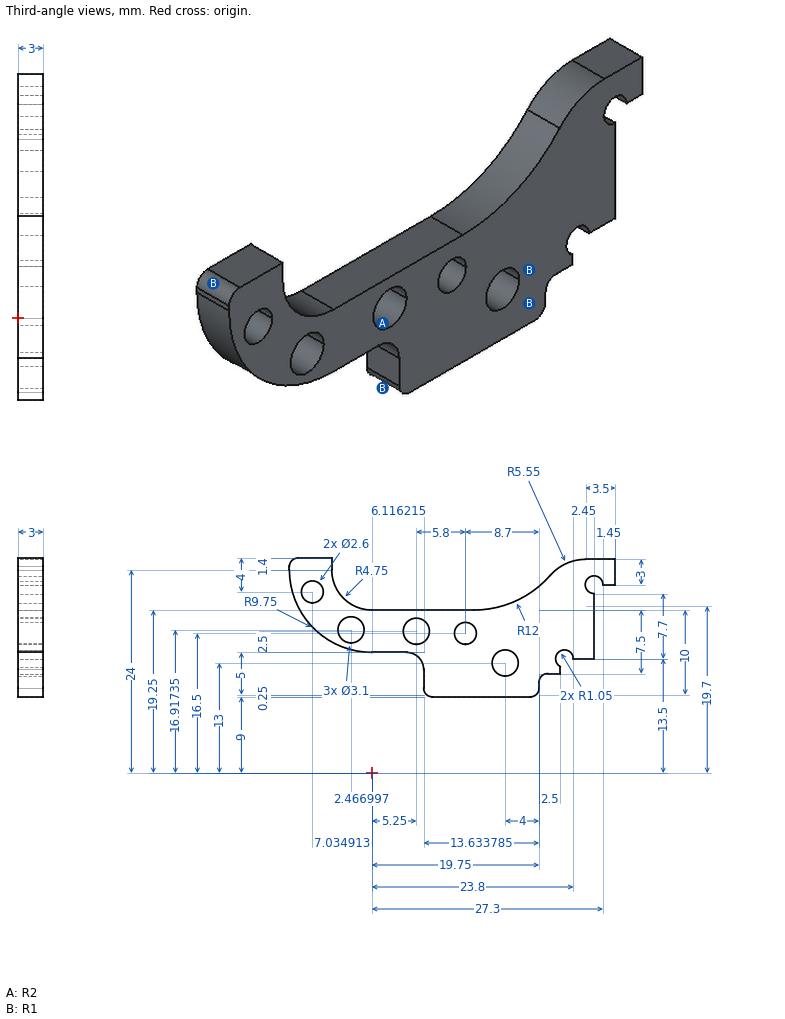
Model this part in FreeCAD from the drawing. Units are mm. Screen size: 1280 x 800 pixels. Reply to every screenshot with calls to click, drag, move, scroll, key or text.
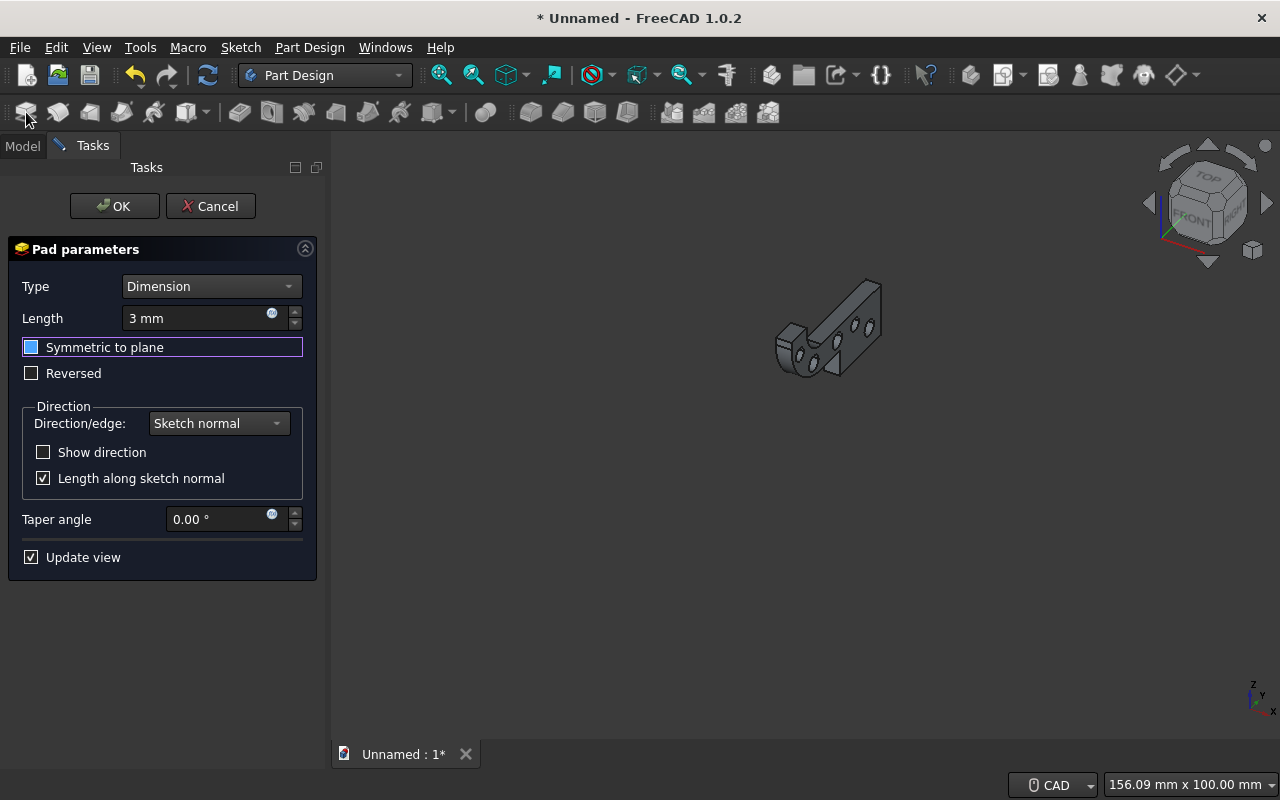
click(115, 206)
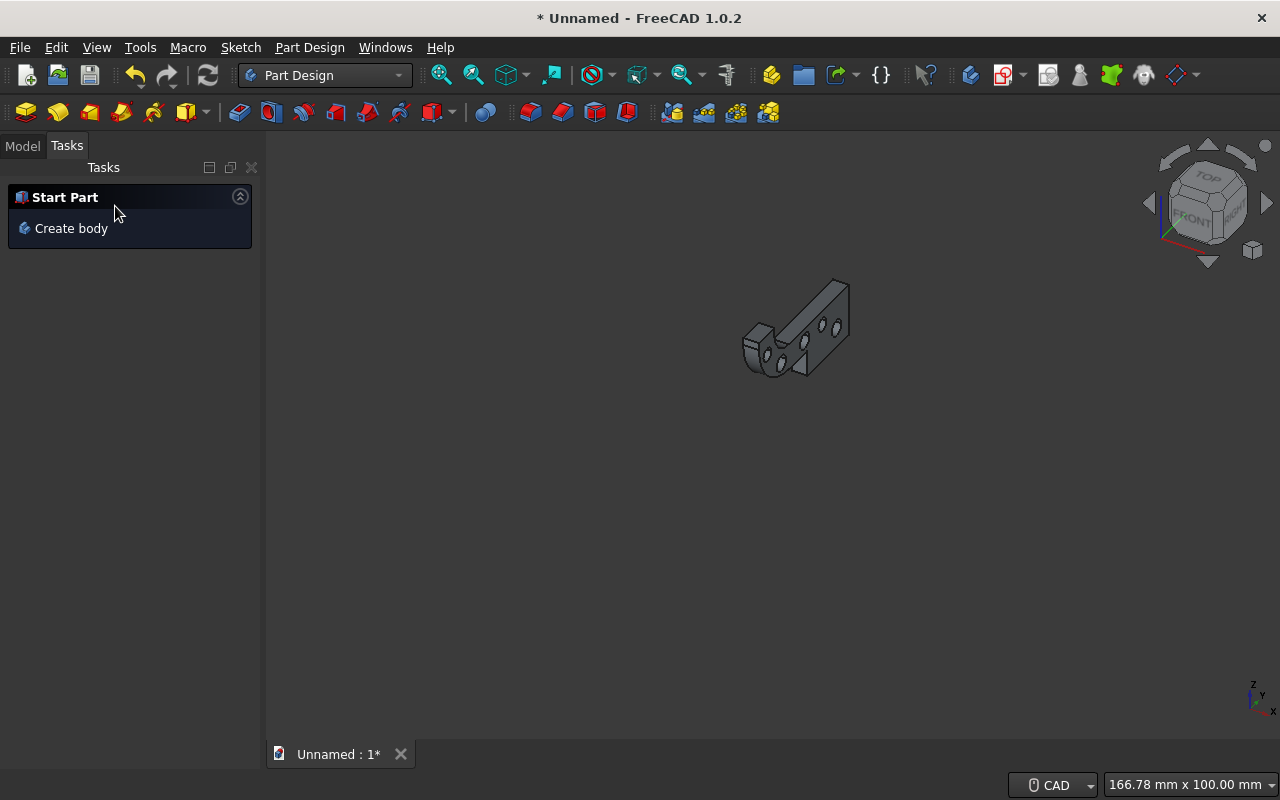
key(v)
key(f)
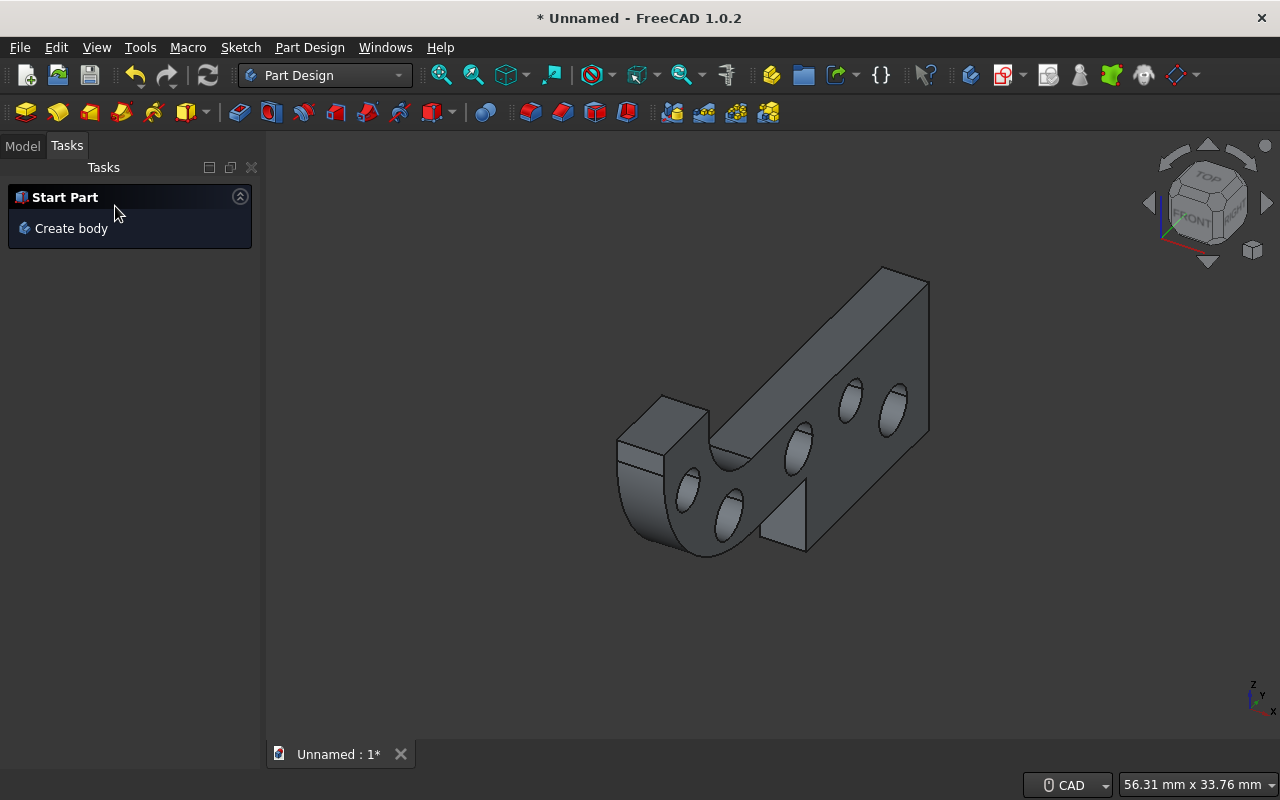
click(834, 472)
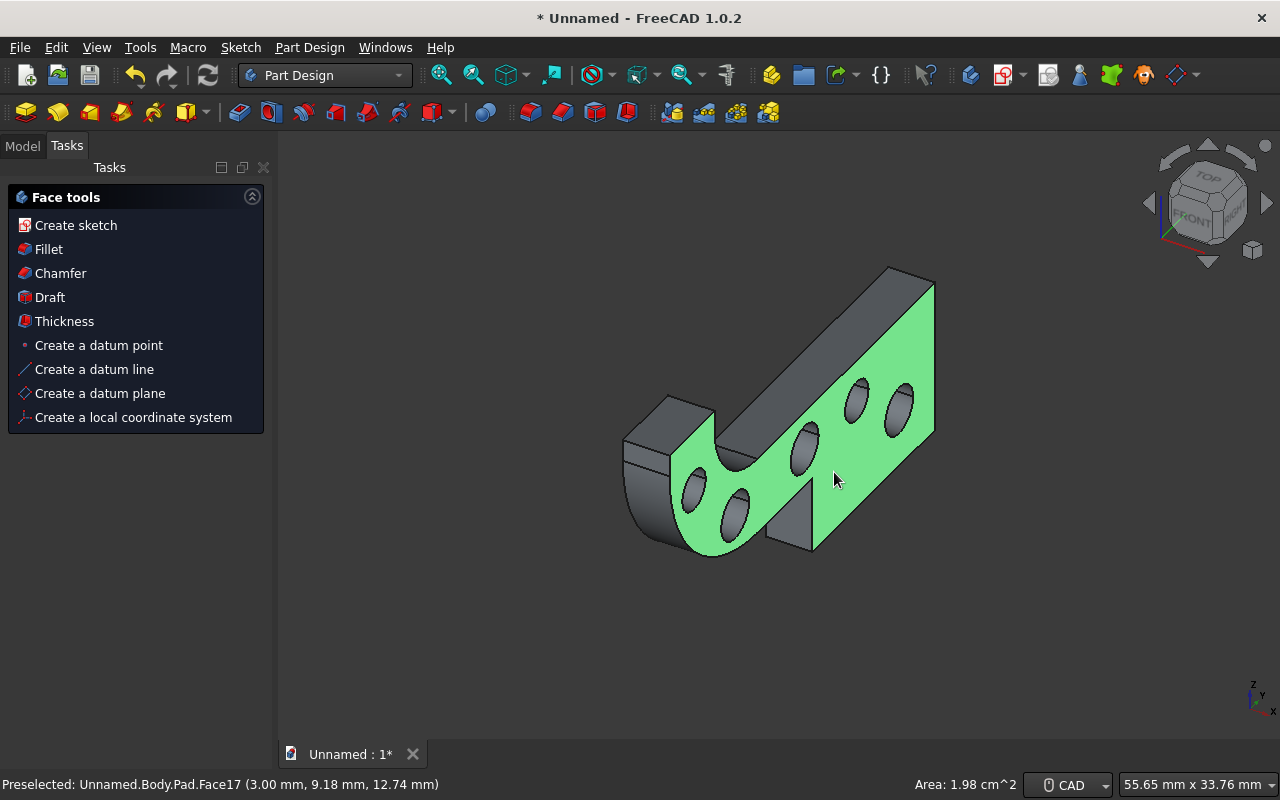
click(1004, 76)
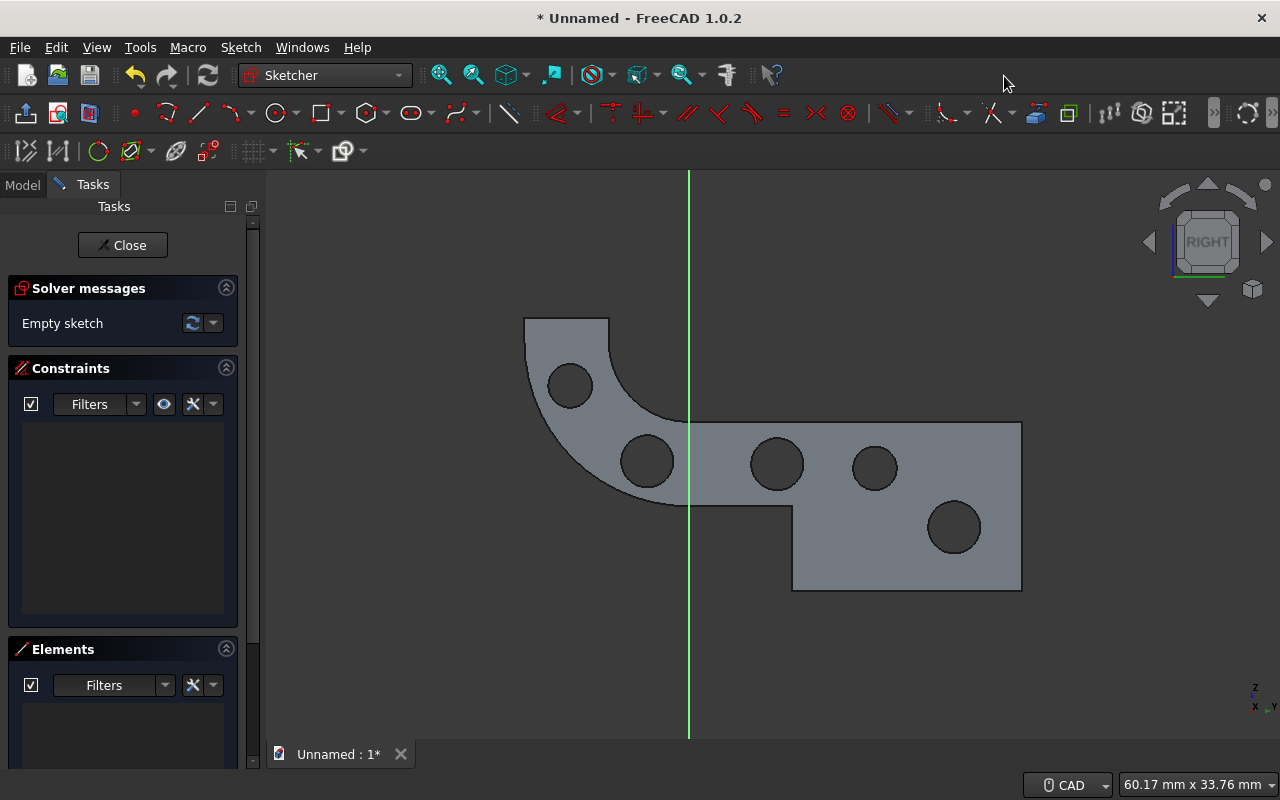
scroll(294, 198, down, 1)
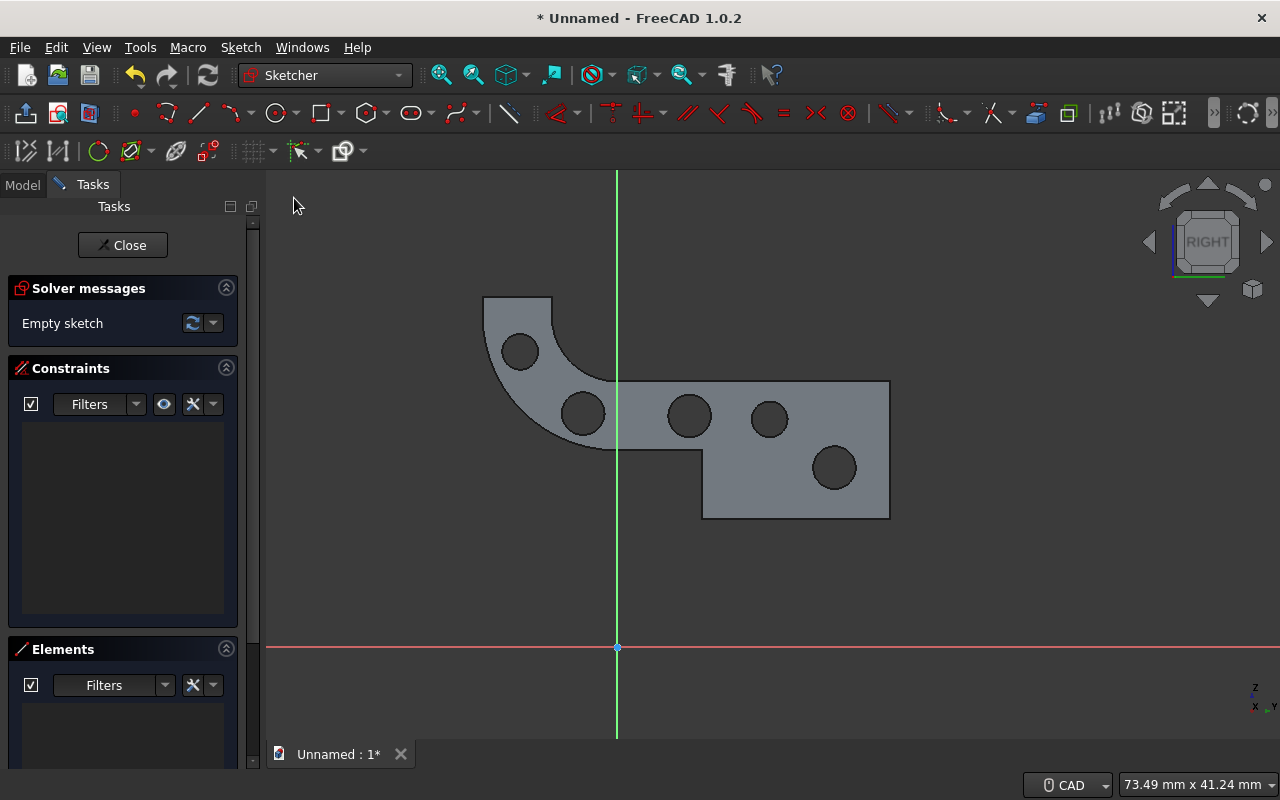
click(168, 114)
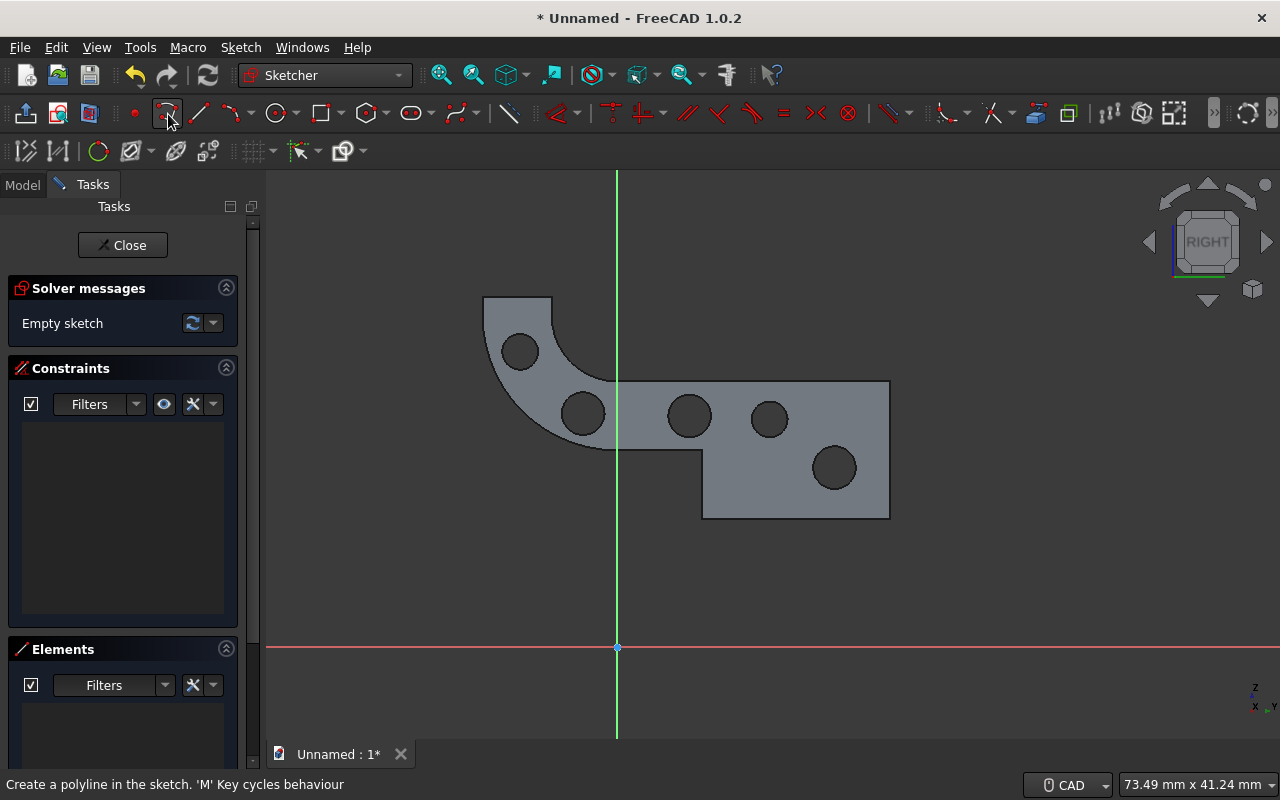
click(946, 461)
click(979, 461)
click(979, 355)
right_click(979, 355)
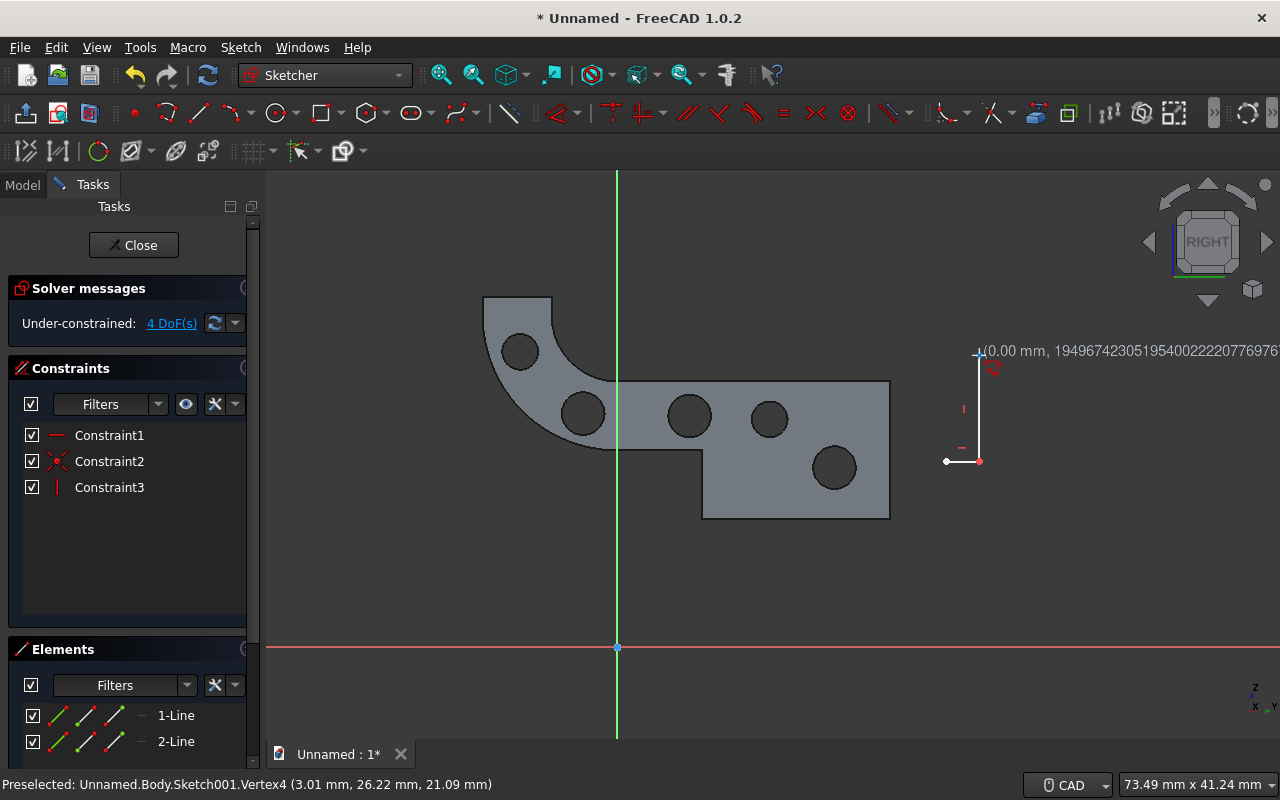
click(994, 340)
click(1014, 340)
click(1014, 299)
click(966, 299)
right_click(966, 299)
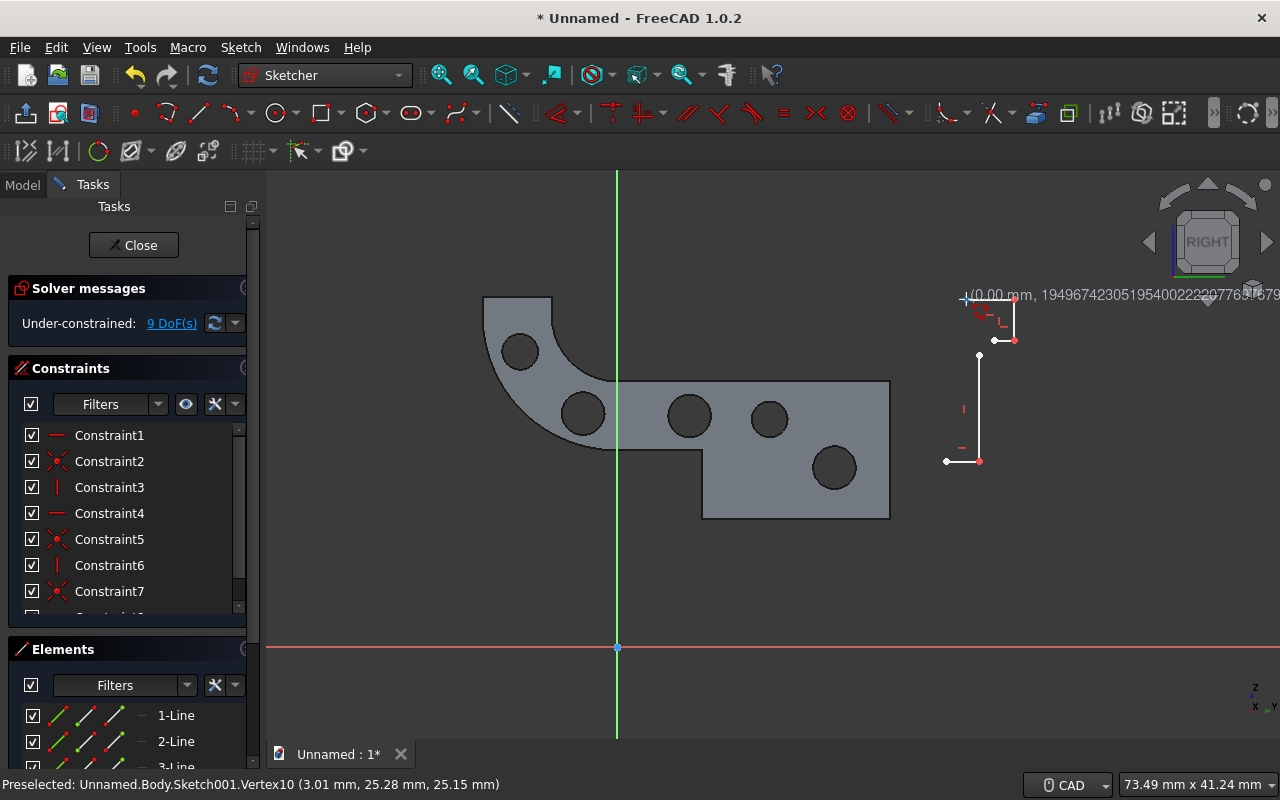
click(783, 381)
click(890, 381)
click(890, 485)
click(924, 485)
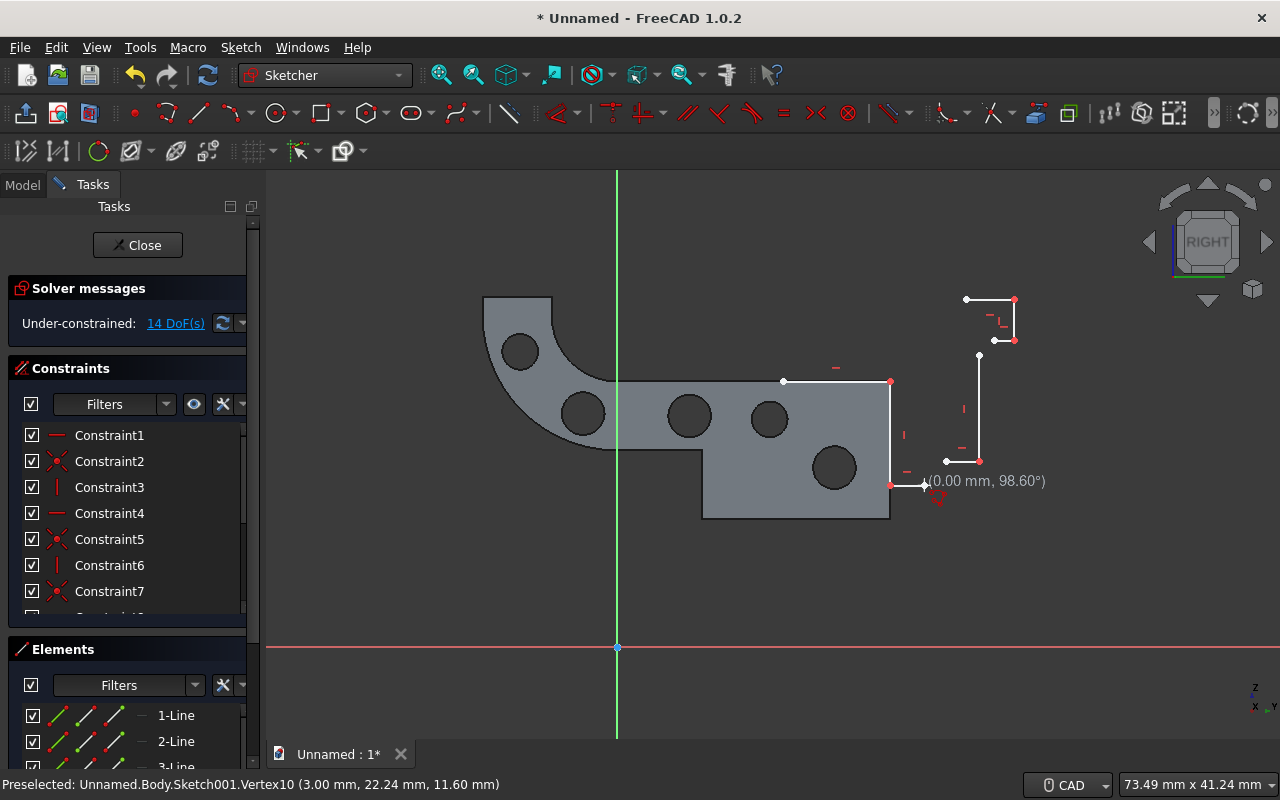
scroll(924, 474, up, 2)